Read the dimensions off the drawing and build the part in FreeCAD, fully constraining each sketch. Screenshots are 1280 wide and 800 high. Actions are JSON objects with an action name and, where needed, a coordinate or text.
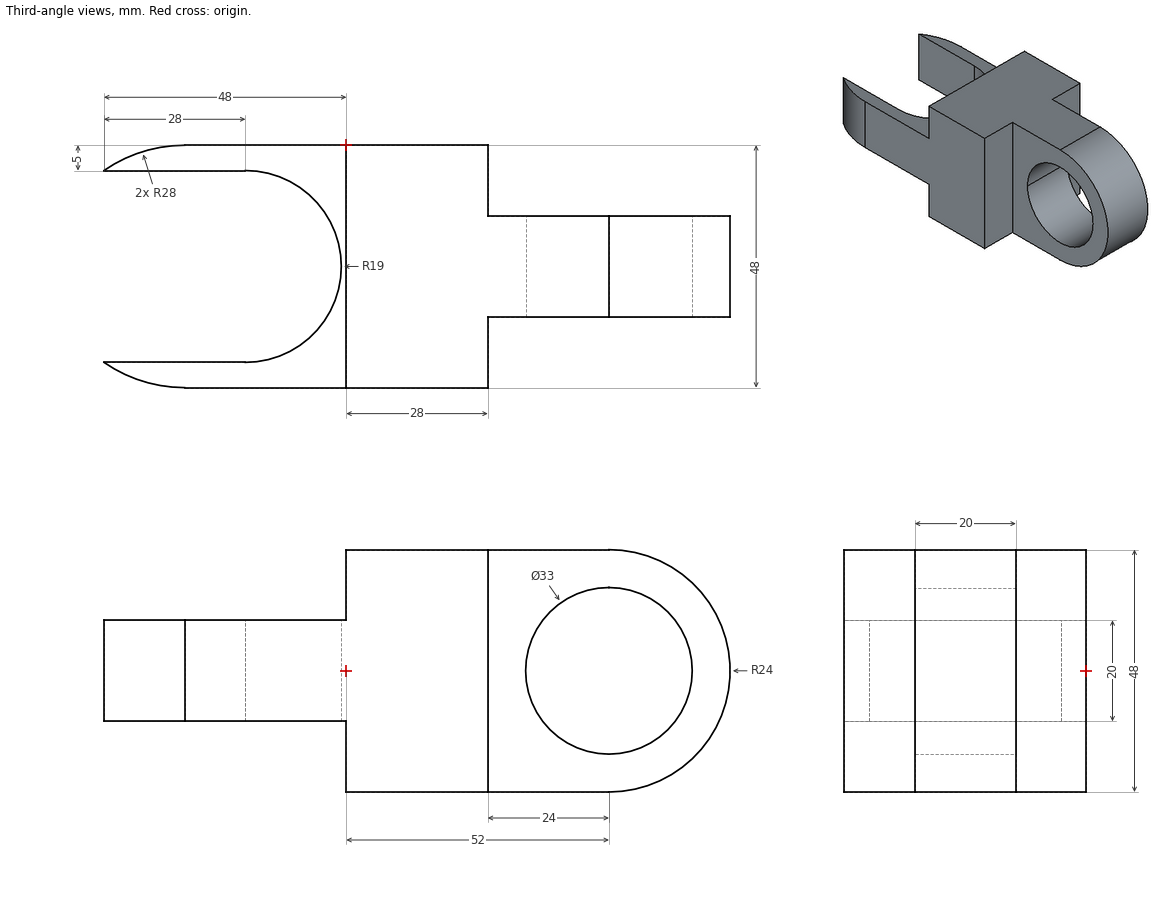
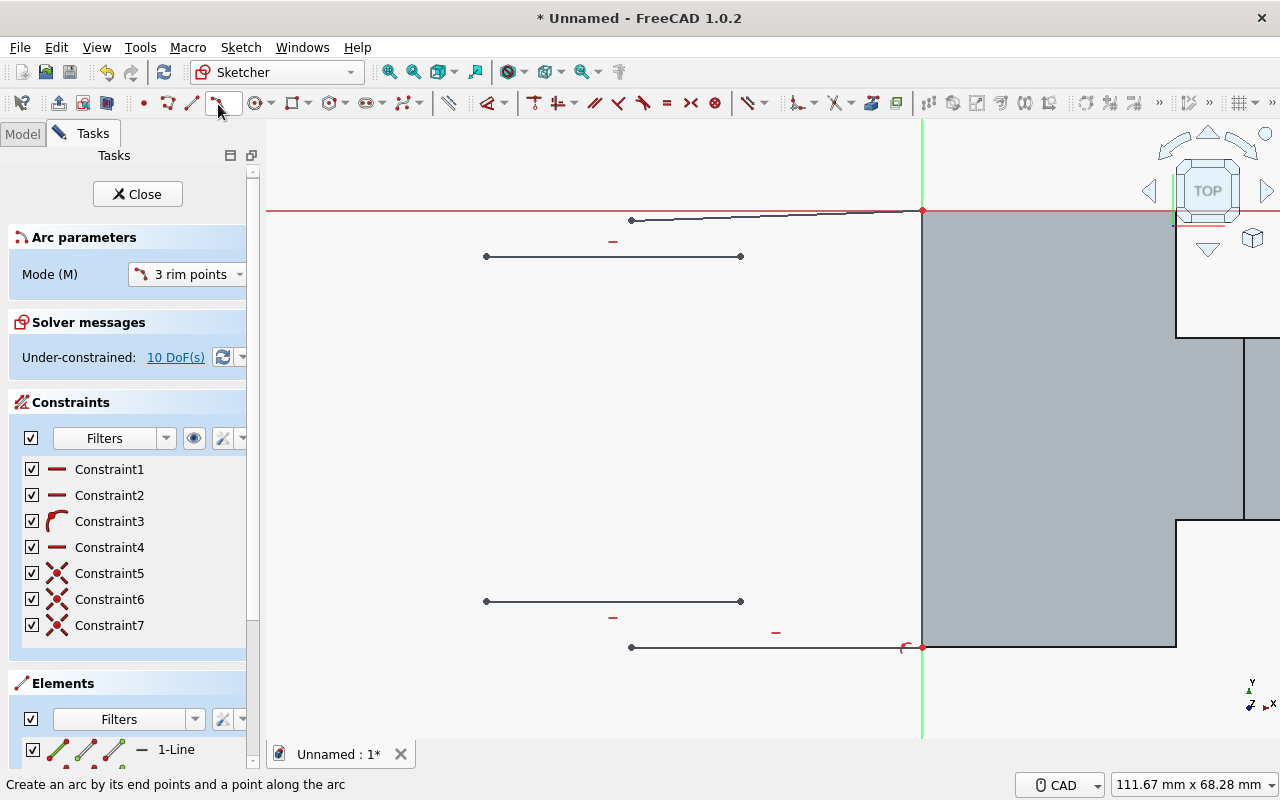
{"action": "left_click", "coordinate": [740, 257]}
{"action": "left_click", "coordinate": [740, 602]}
{"action": "left_click", "coordinate": [905, 482]}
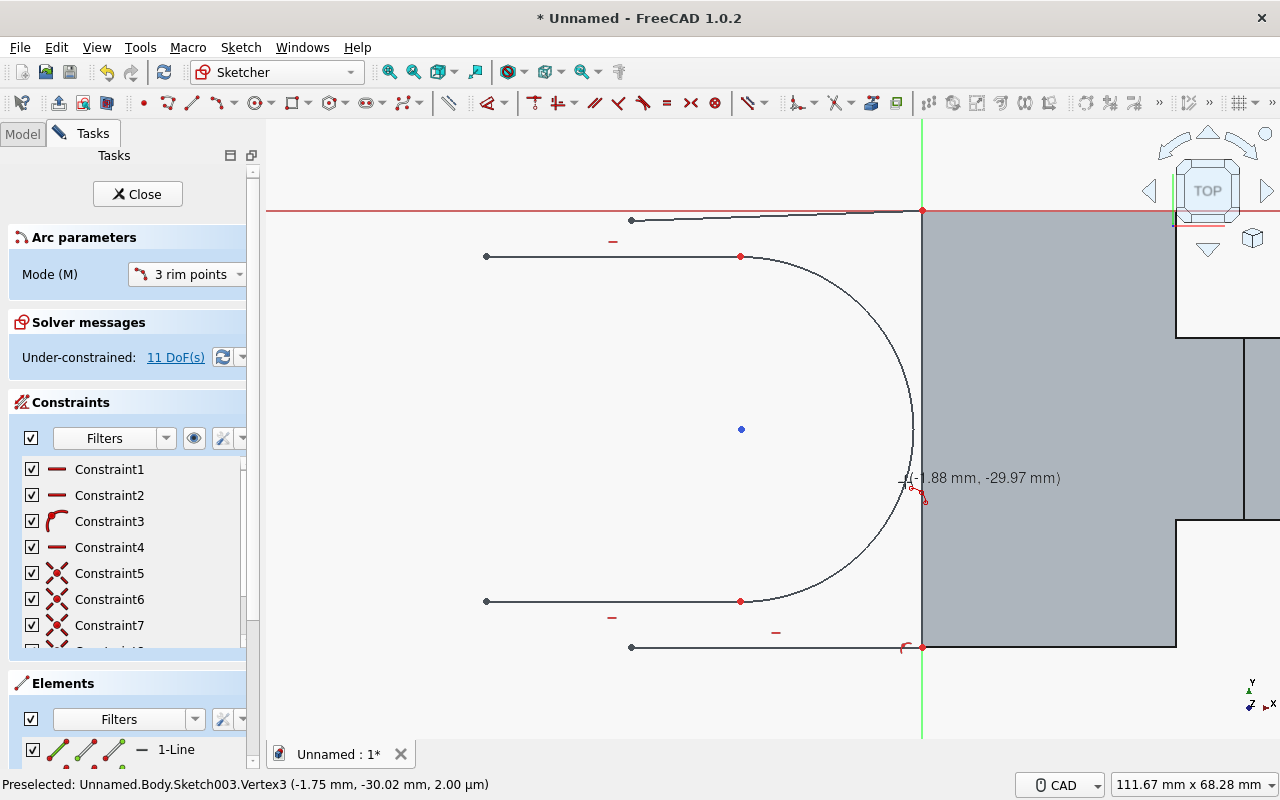
{"action": "left_click", "coordinate": [486, 602]}
{"action": "left_click", "coordinate": [631, 648]}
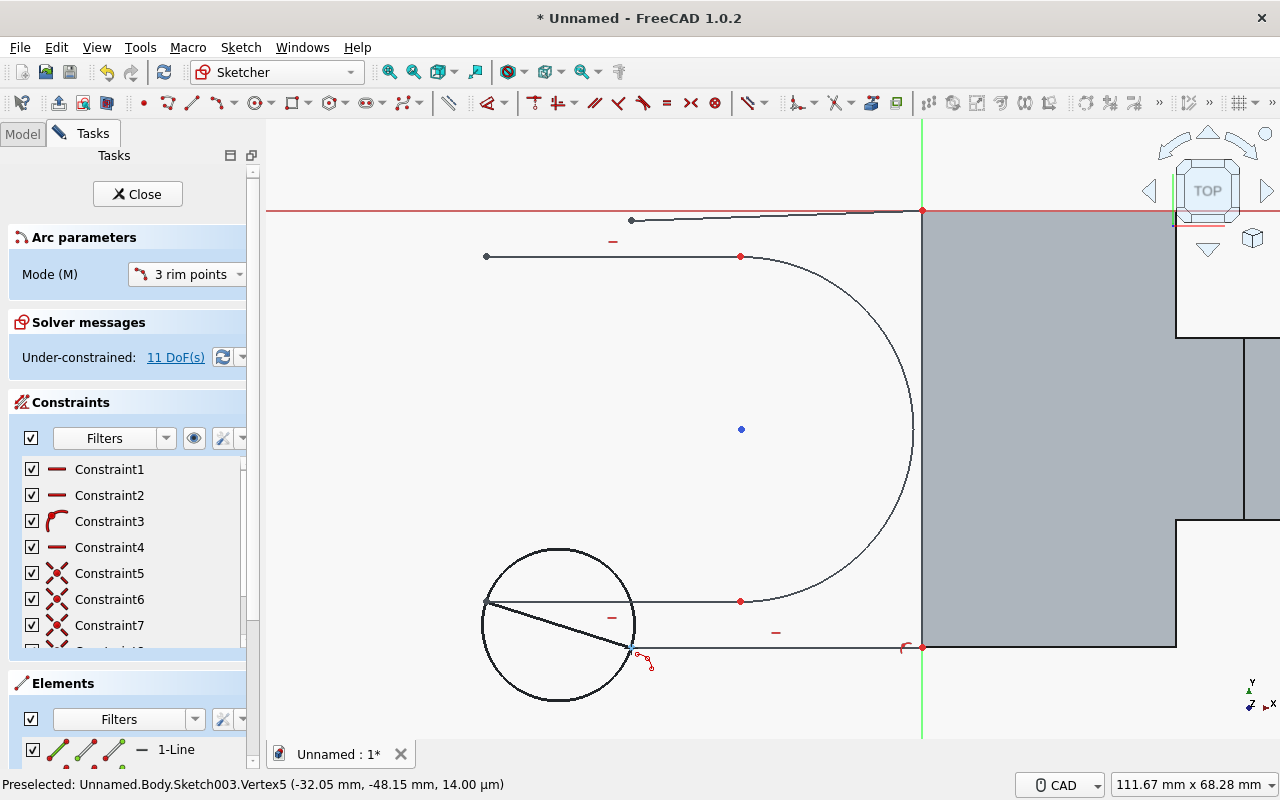
{"action": "scroll", "coordinate": [555, 635], "scroll_direction": "up", "scroll_amount": 2}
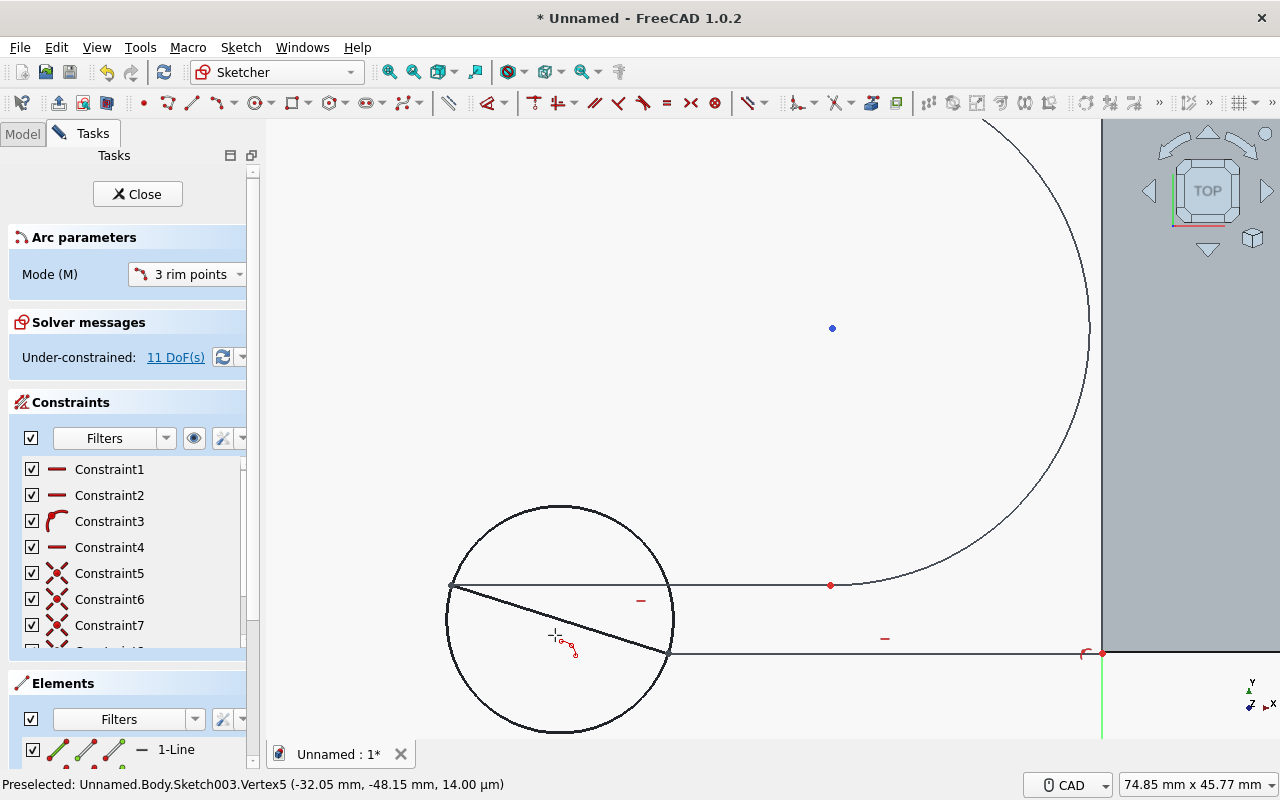
{"action": "left_click", "coordinate": [555, 635]}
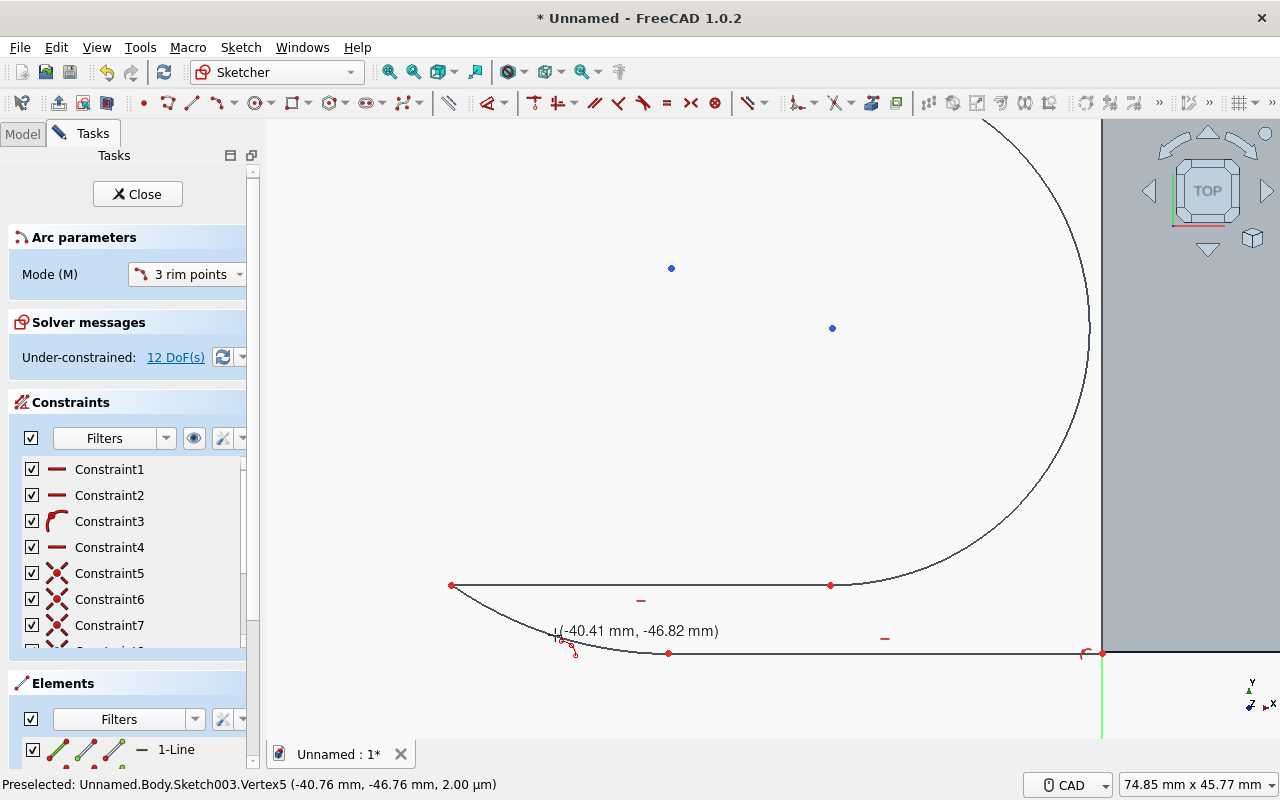
{"action": "scroll", "coordinate": [556, 637], "scroll_direction": "down", "scroll_amount": 2}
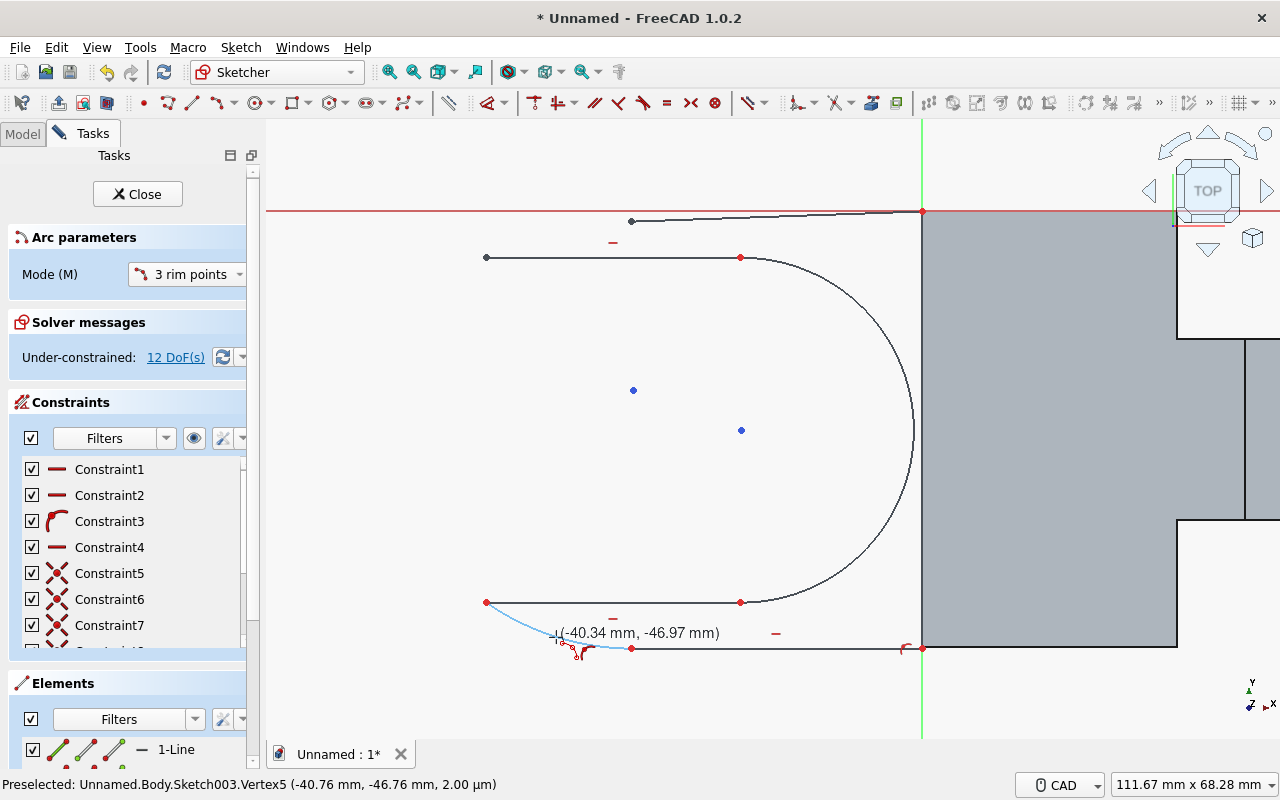
{"action": "left_click", "coordinate": [631, 222]}
{"action": "left_click", "coordinate": [486, 258]}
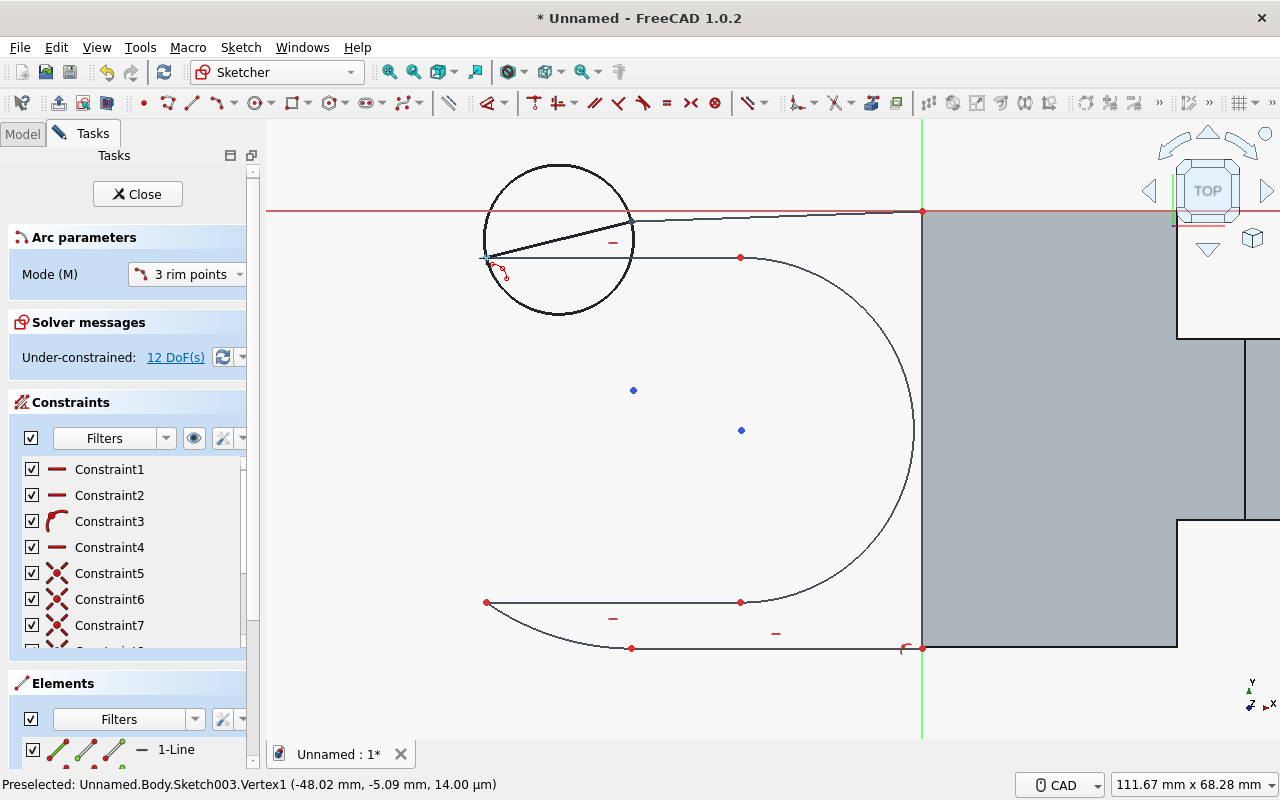
{"action": "scroll", "coordinate": [556, 223], "scroll_direction": "up", "scroll_amount": 2}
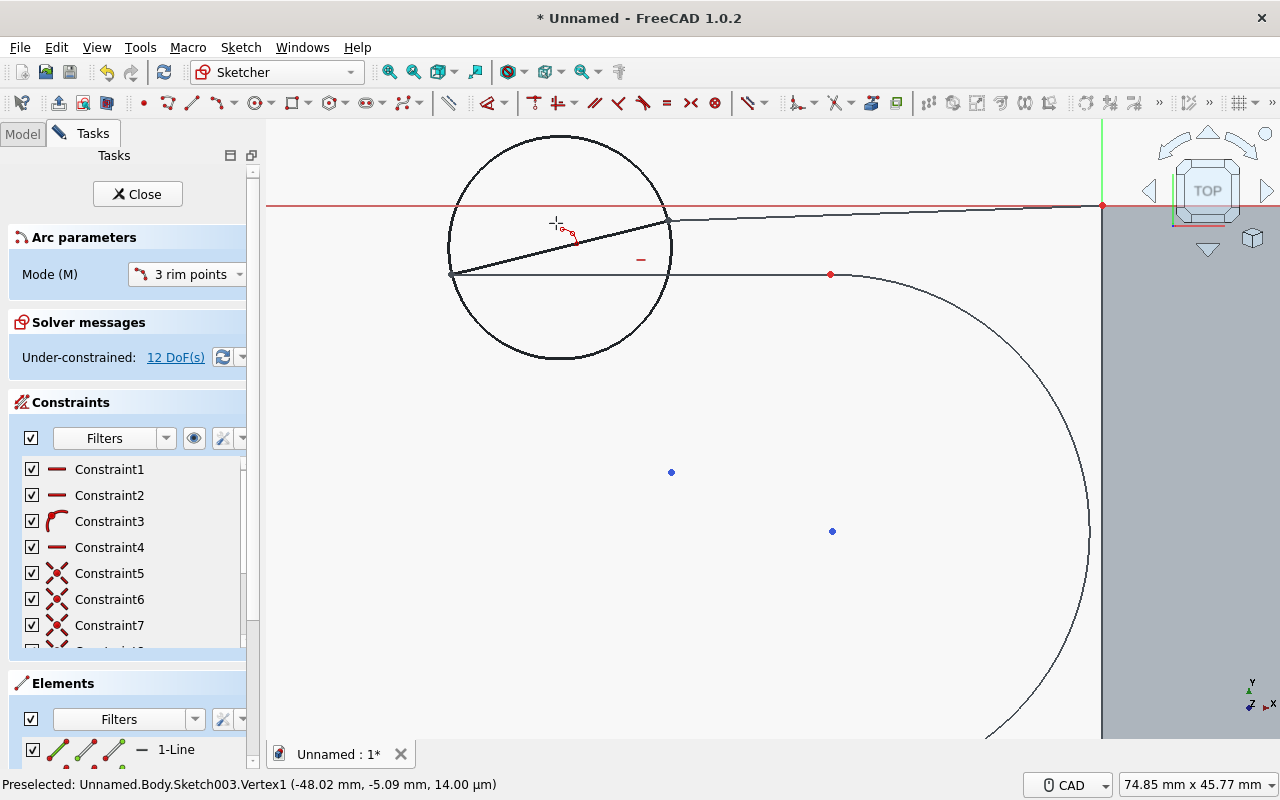
{"action": "left_click", "coordinate": [555, 223]}
{"action": "key", "text": "Escape"}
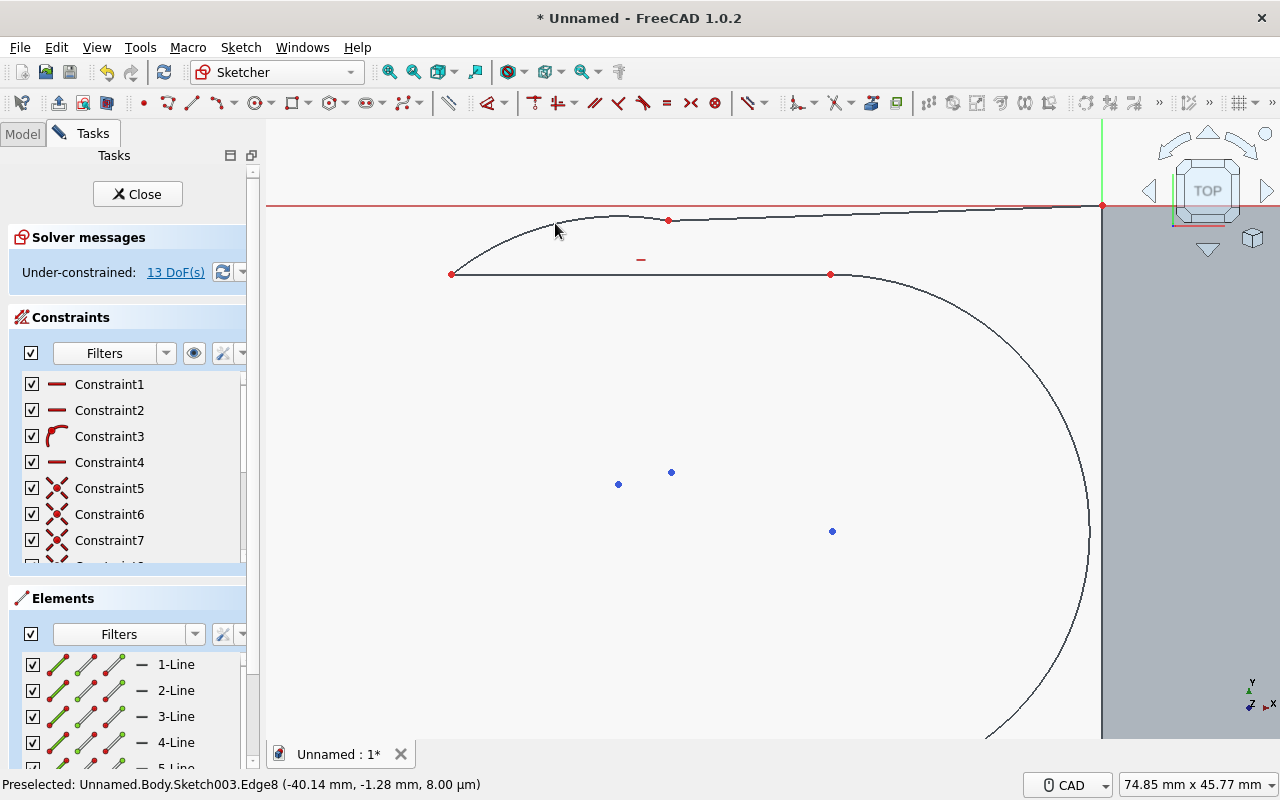
{"action": "left_click", "coordinate": [566, 275]}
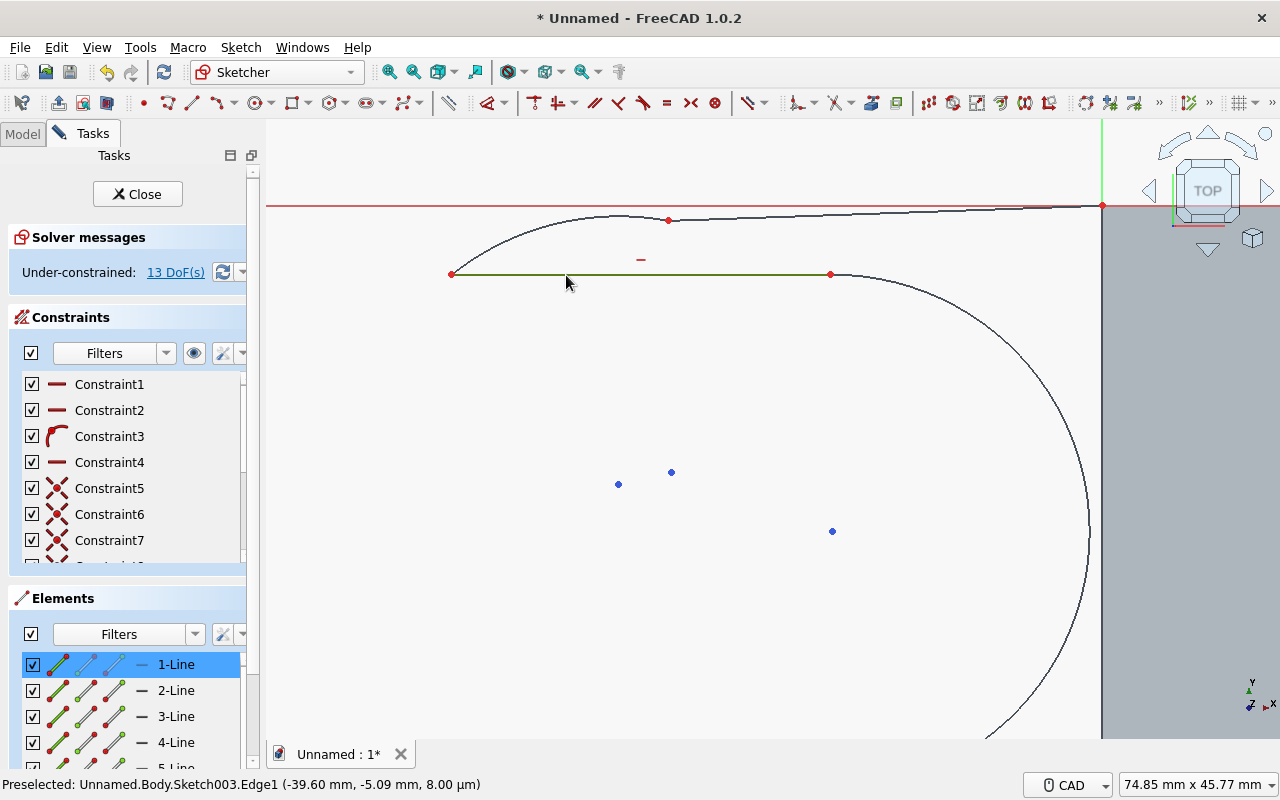
{"action": "left_click", "coordinate": [1040, 684]}